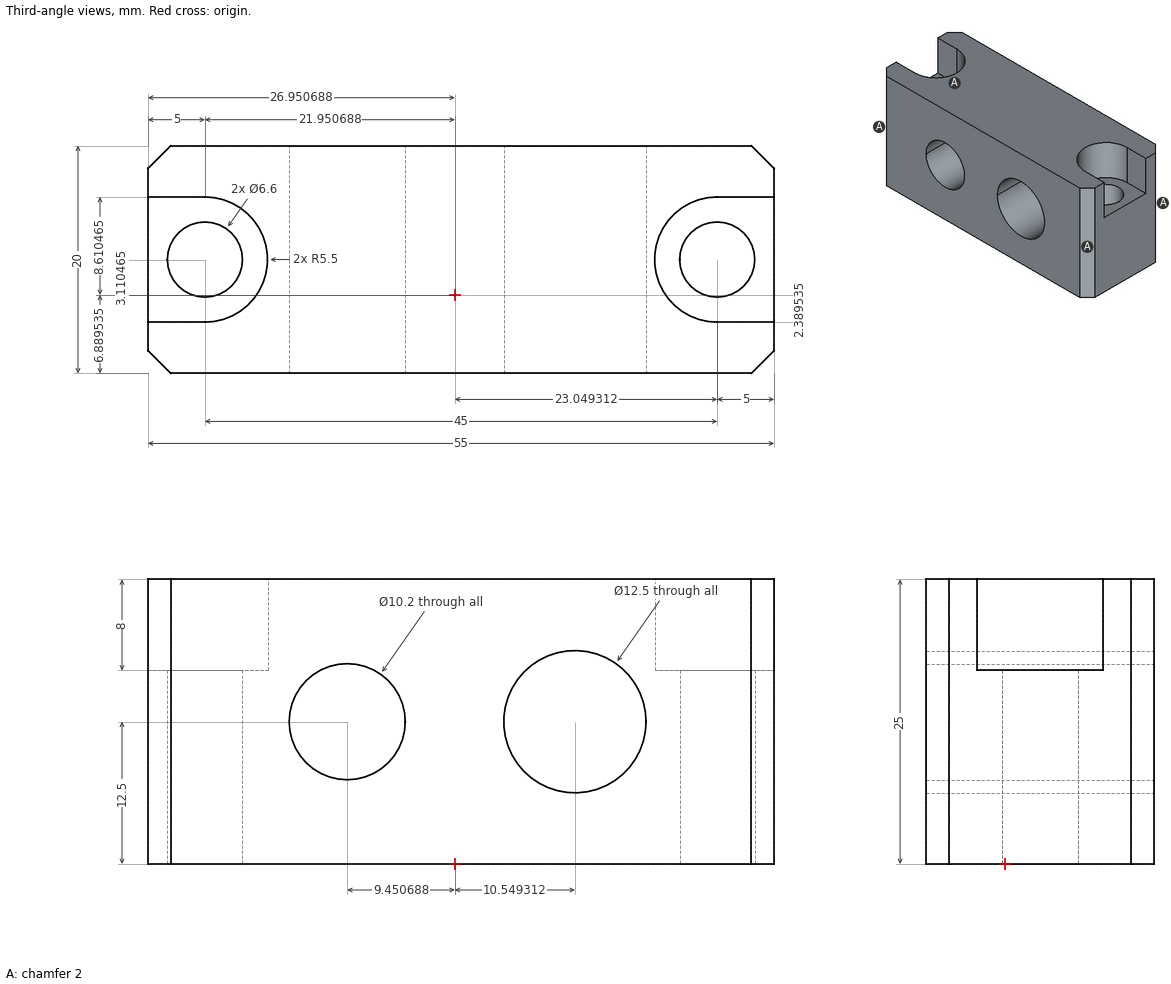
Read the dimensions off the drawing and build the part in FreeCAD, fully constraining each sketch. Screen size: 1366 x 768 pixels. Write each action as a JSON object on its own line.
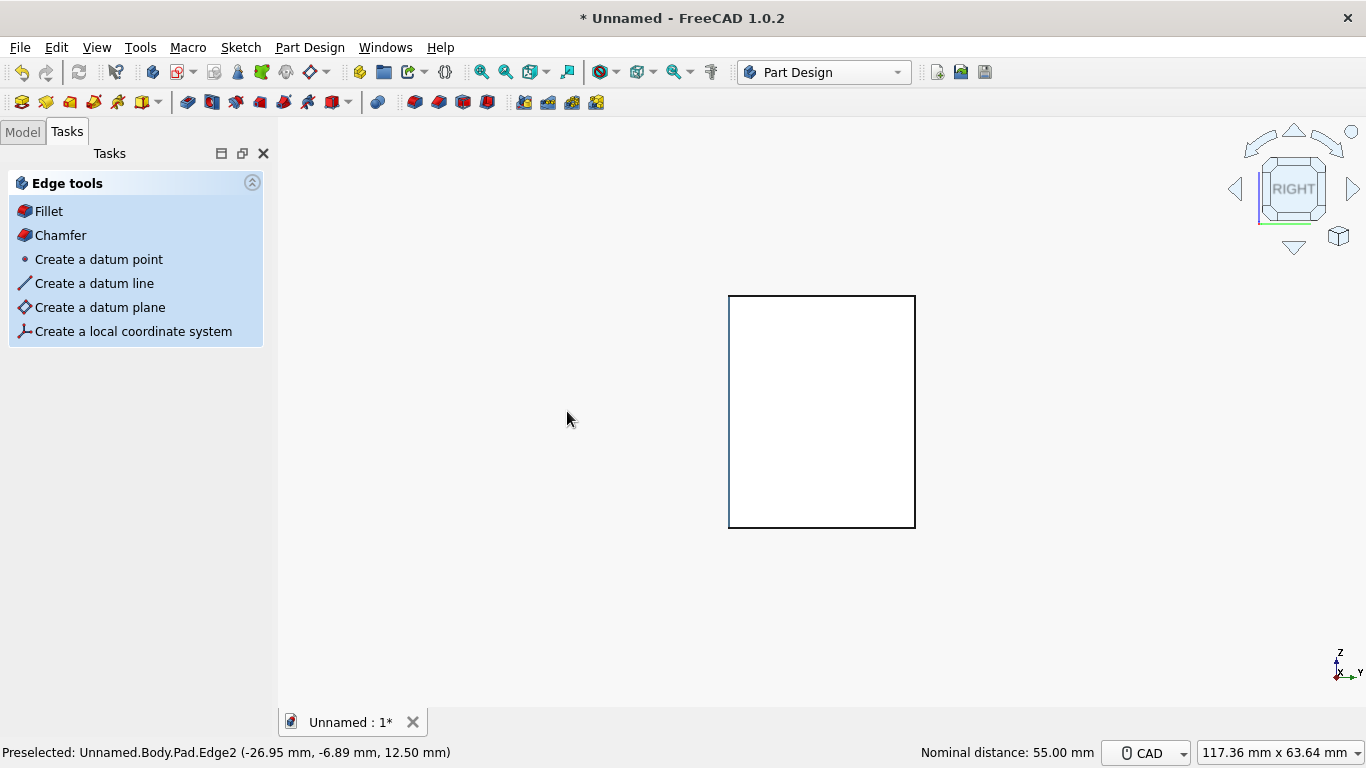
{"action": "left_click", "coordinate": [482, 72]}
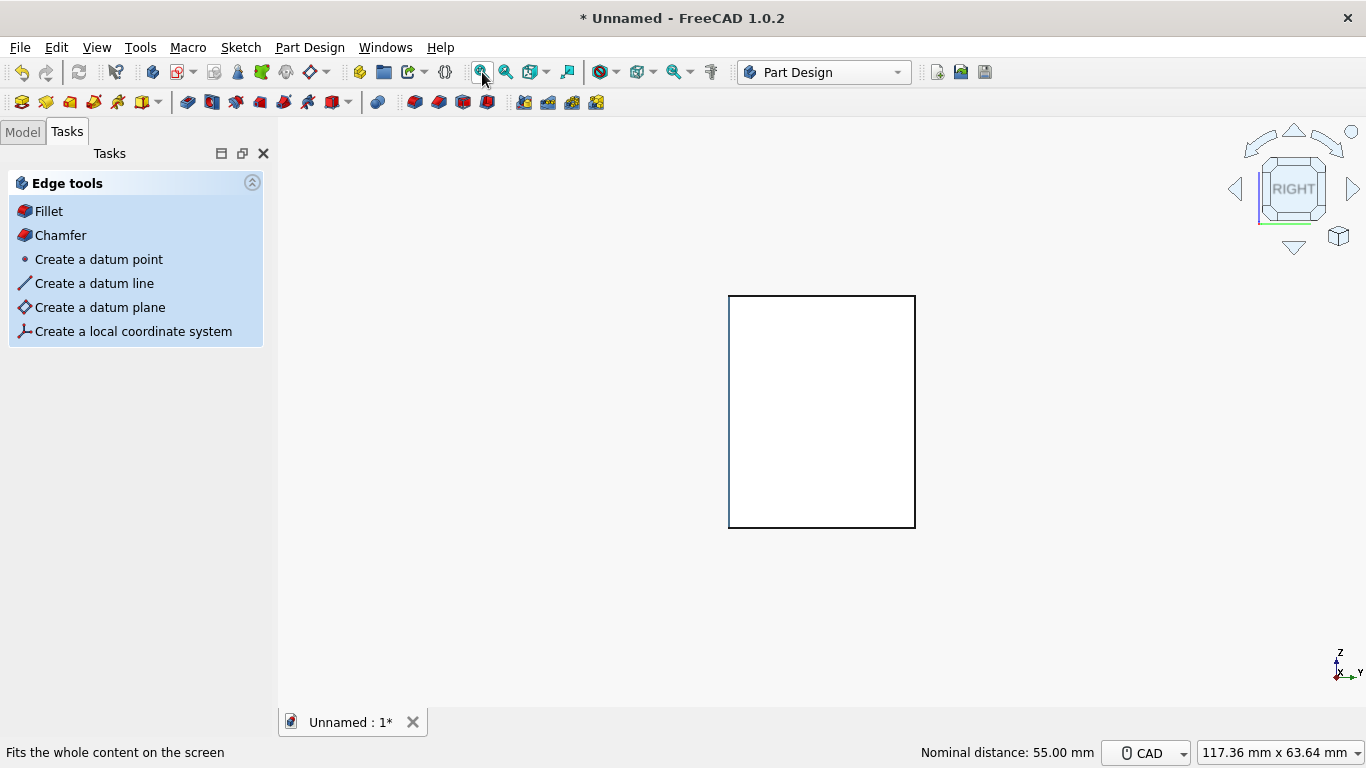
{"action": "left_click", "coordinate": [915, 411], "text": "ctrl"}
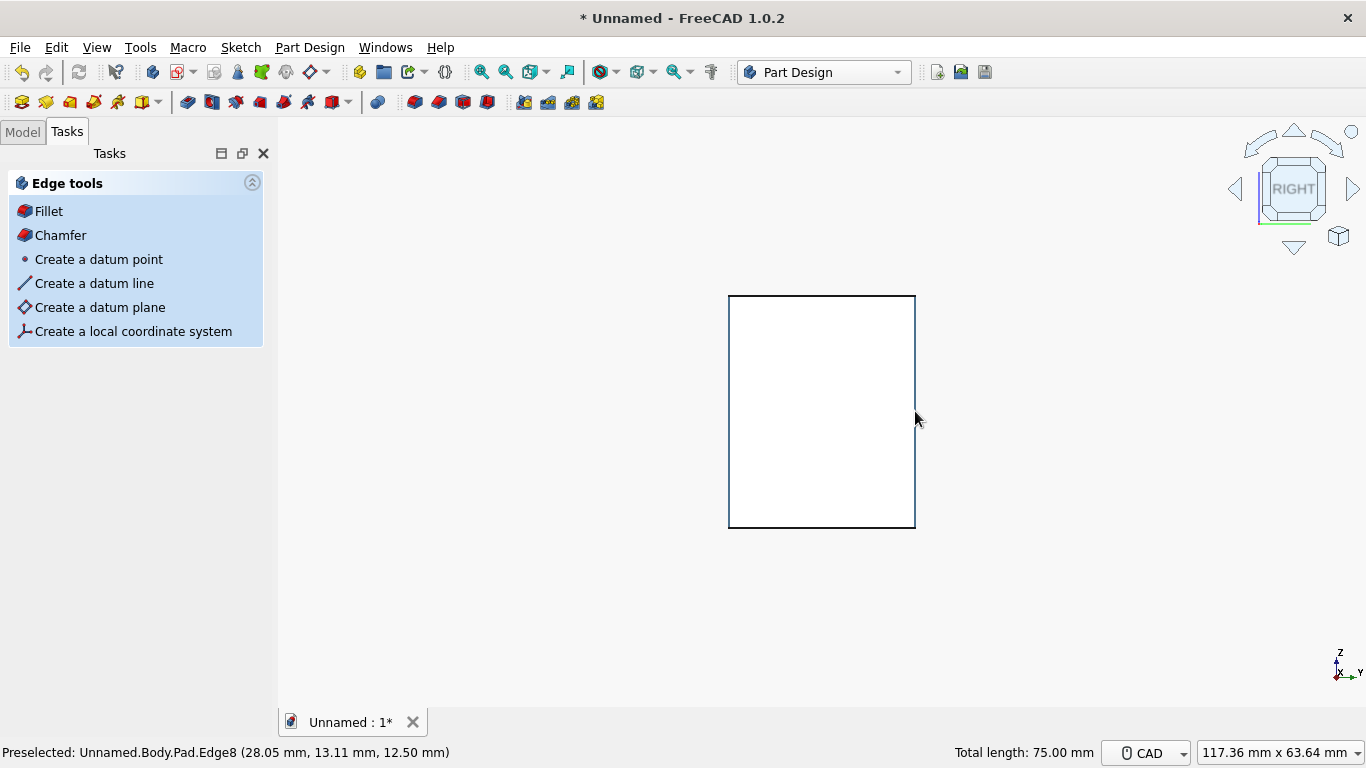
{"action": "key", "text": "5"}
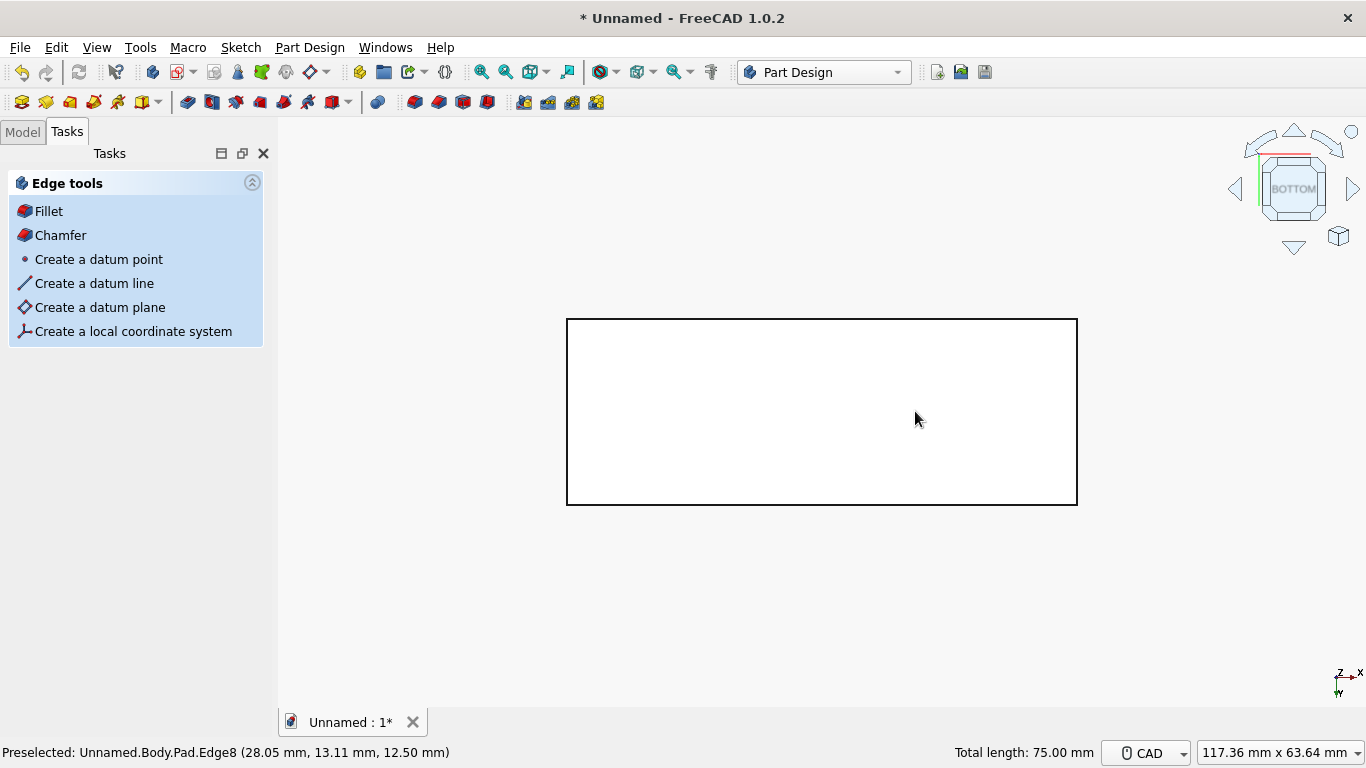
{"action": "key", "text": "4"}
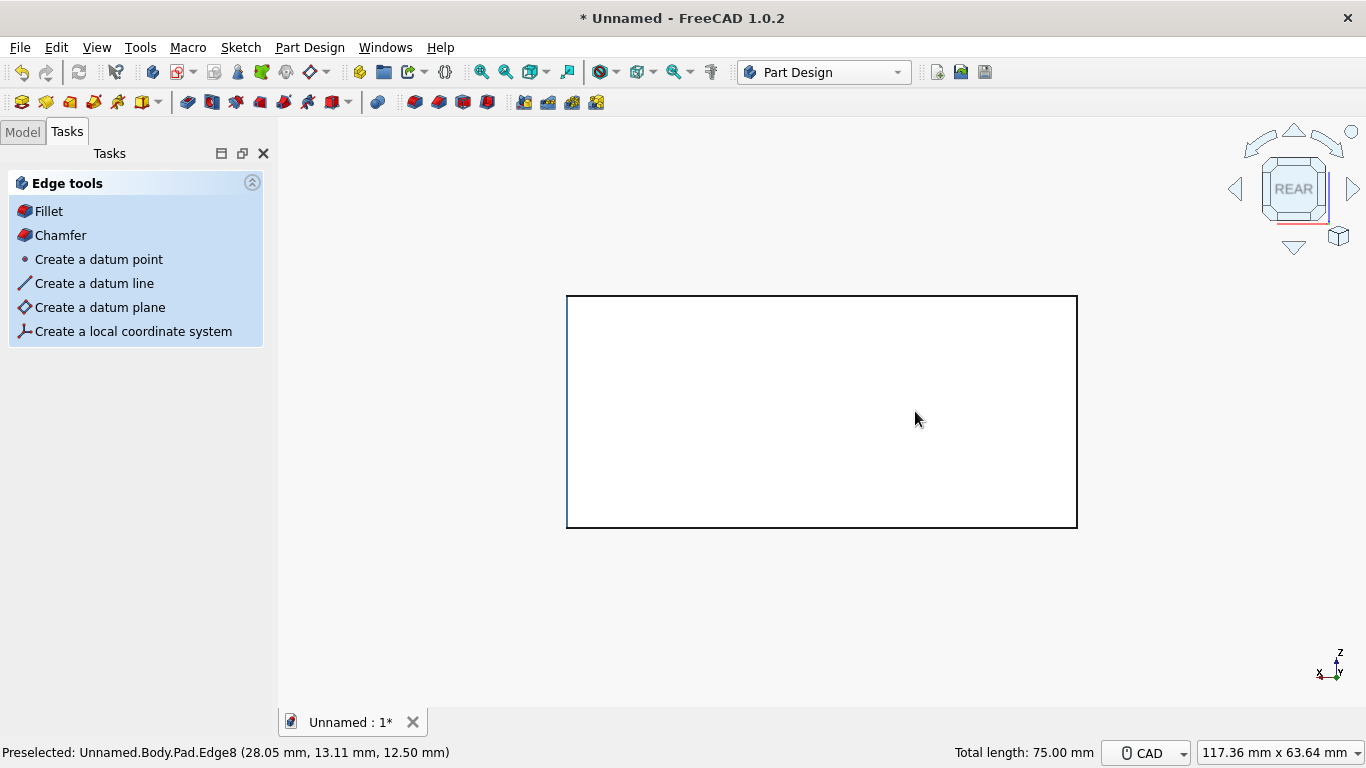
{"action": "left_click", "coordinate": [1077, 411], "text": "ctrl"}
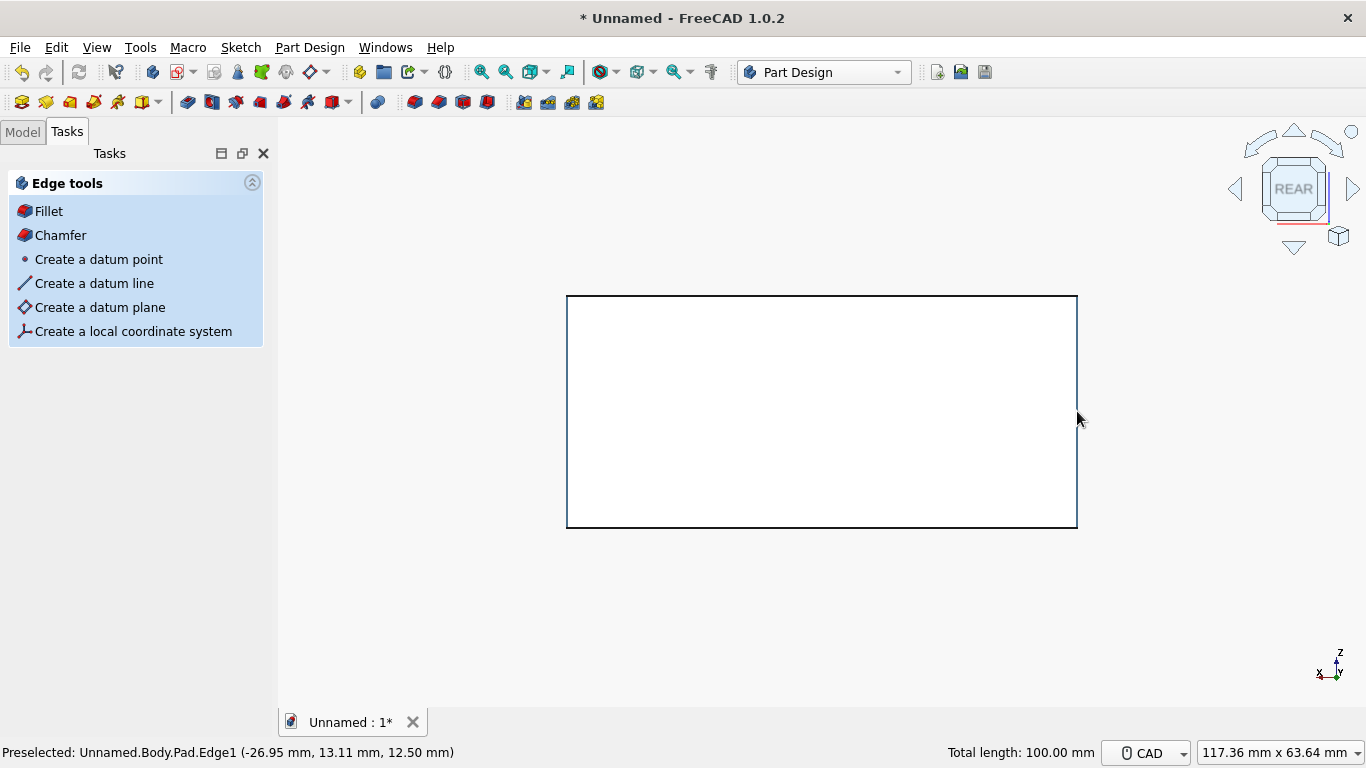
{"action": "left_click", "coordinate": [440, 102]}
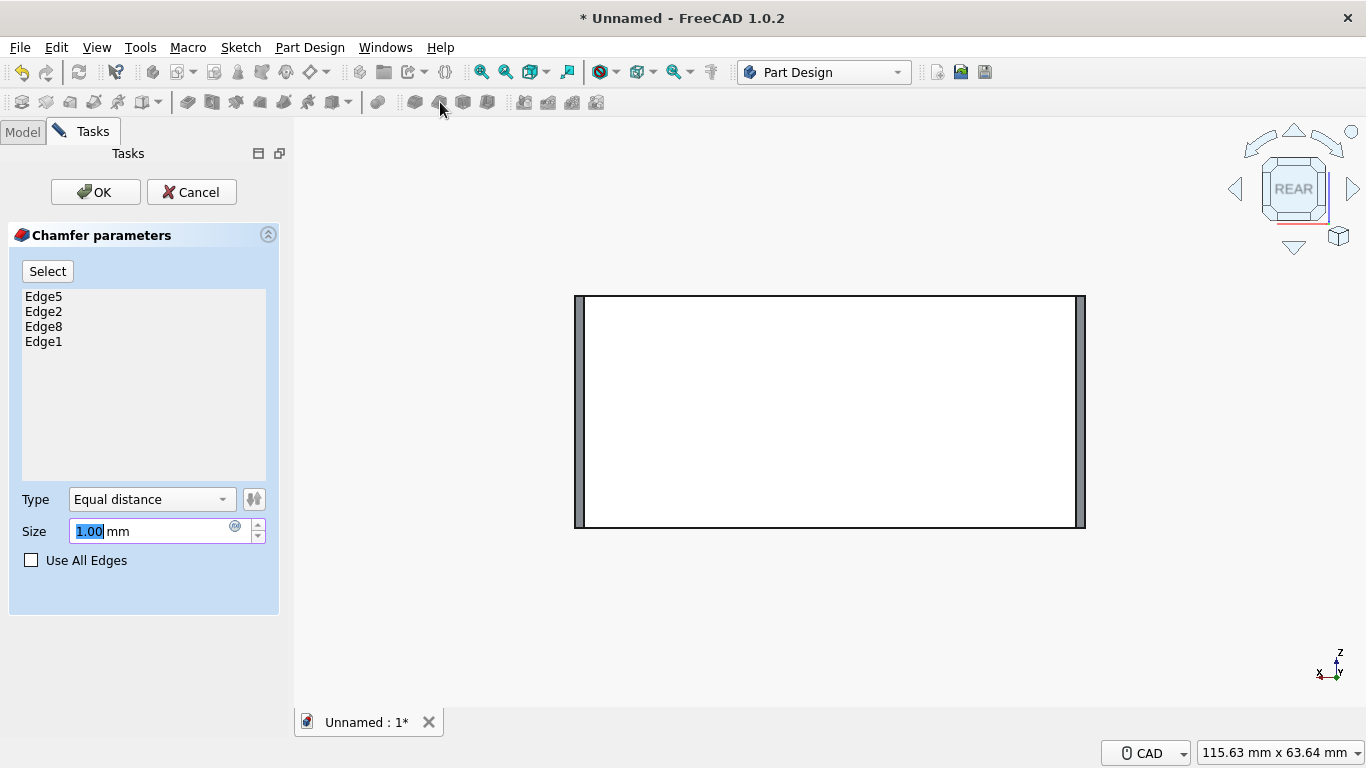
{"action": "type", "text": "2"}
{"action": "key", "text": "Tab"}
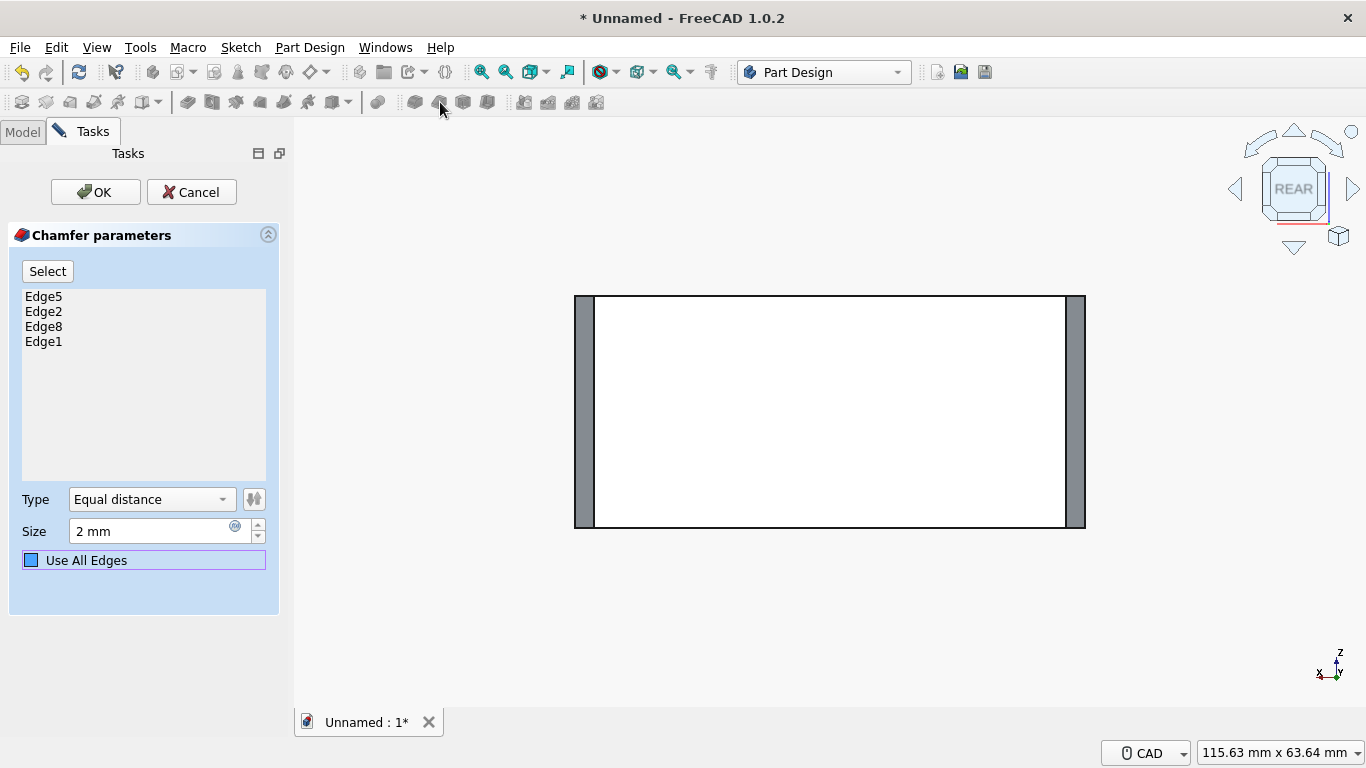
{"action": "left_click", "coordinate": [96, 192]}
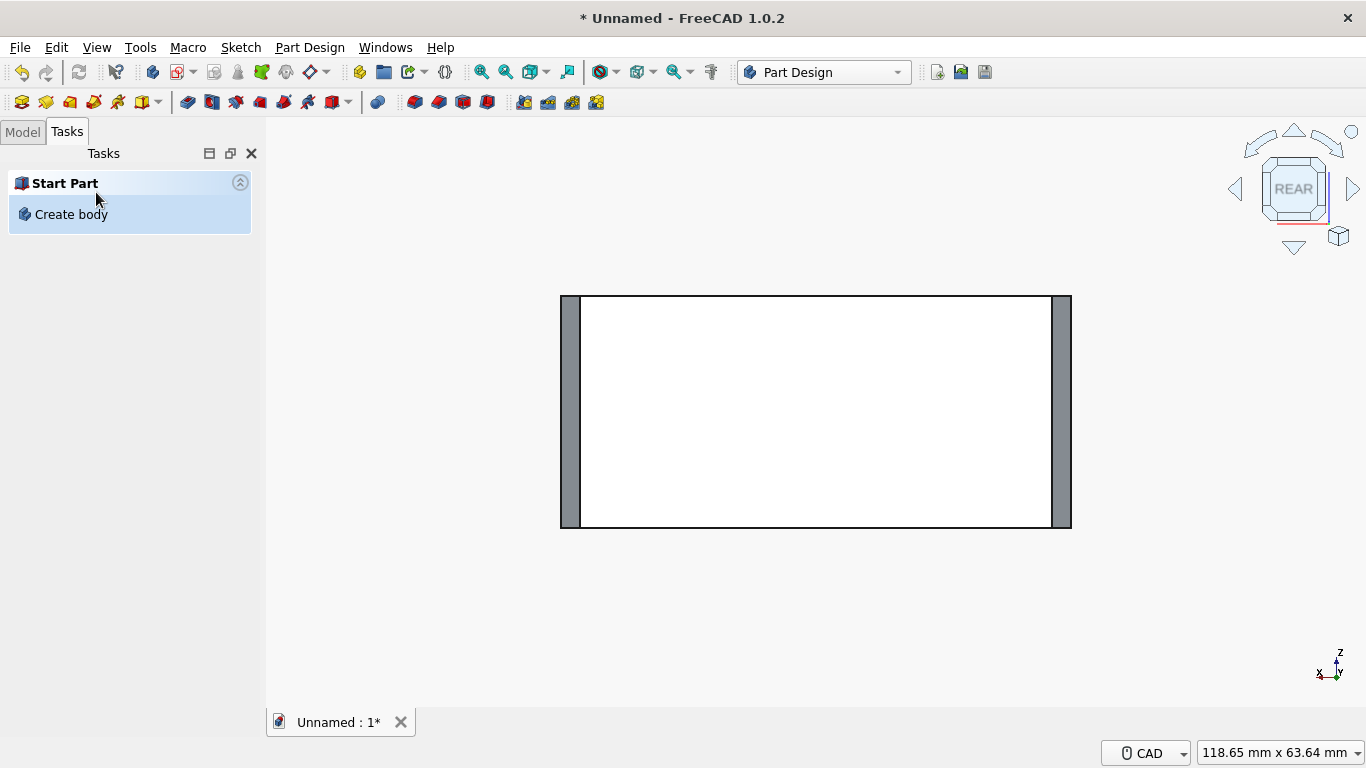
{"action": "key", "text": "0"}